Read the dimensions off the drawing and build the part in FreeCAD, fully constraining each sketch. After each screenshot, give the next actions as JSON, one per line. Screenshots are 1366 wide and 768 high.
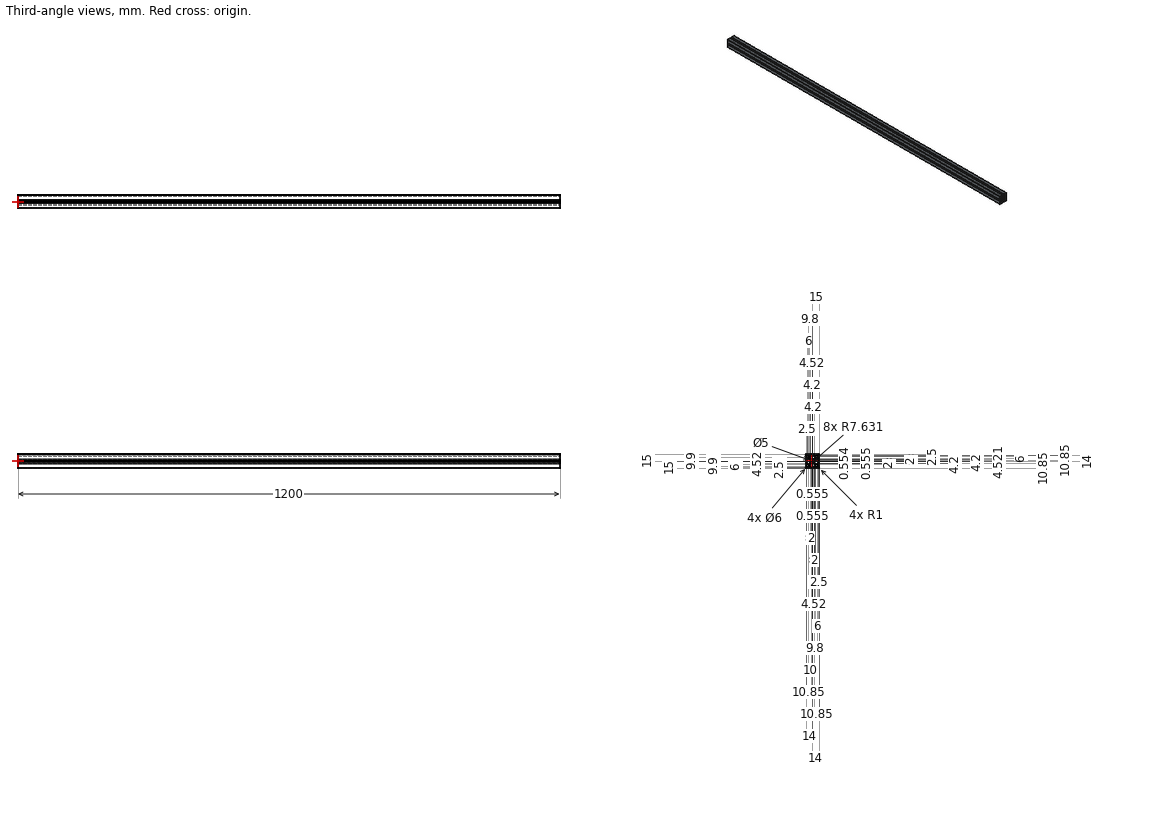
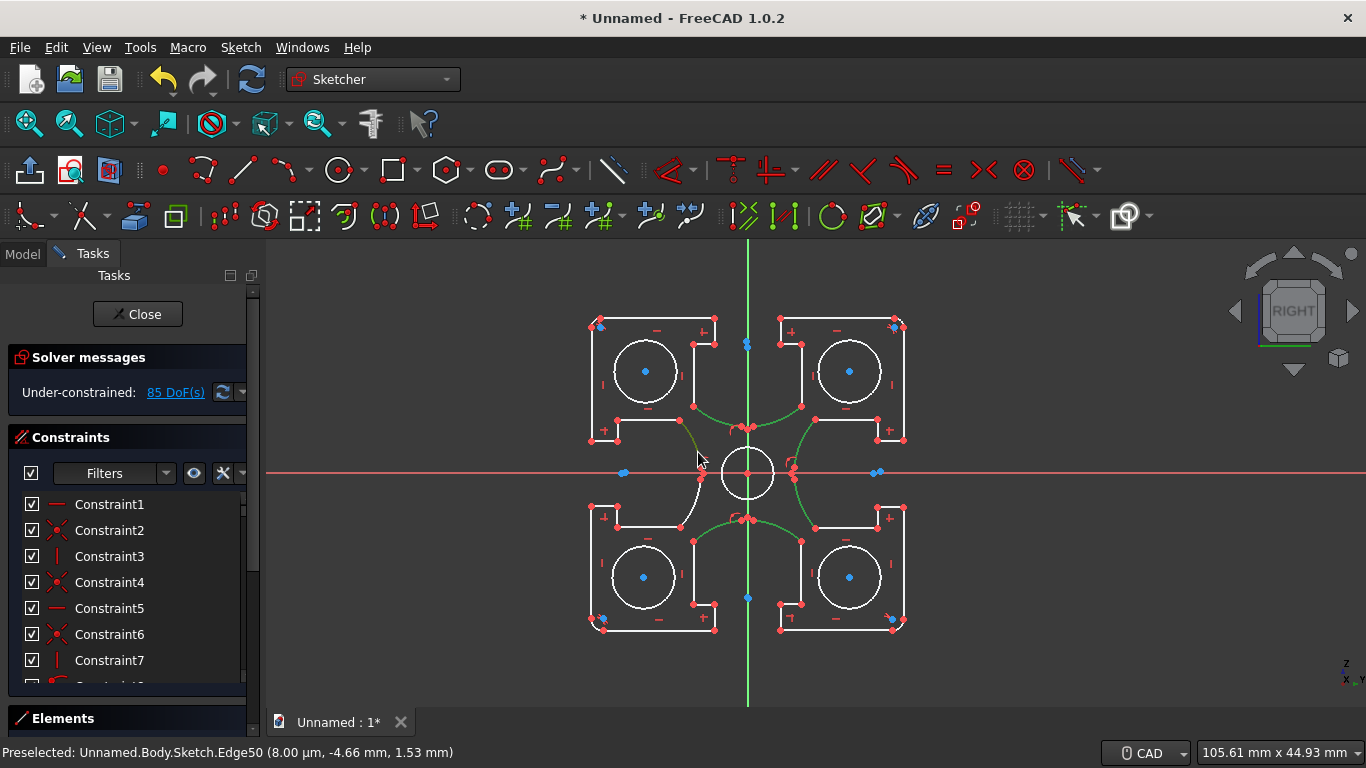
{"action": "left_click", "coordinate": [690, 514]}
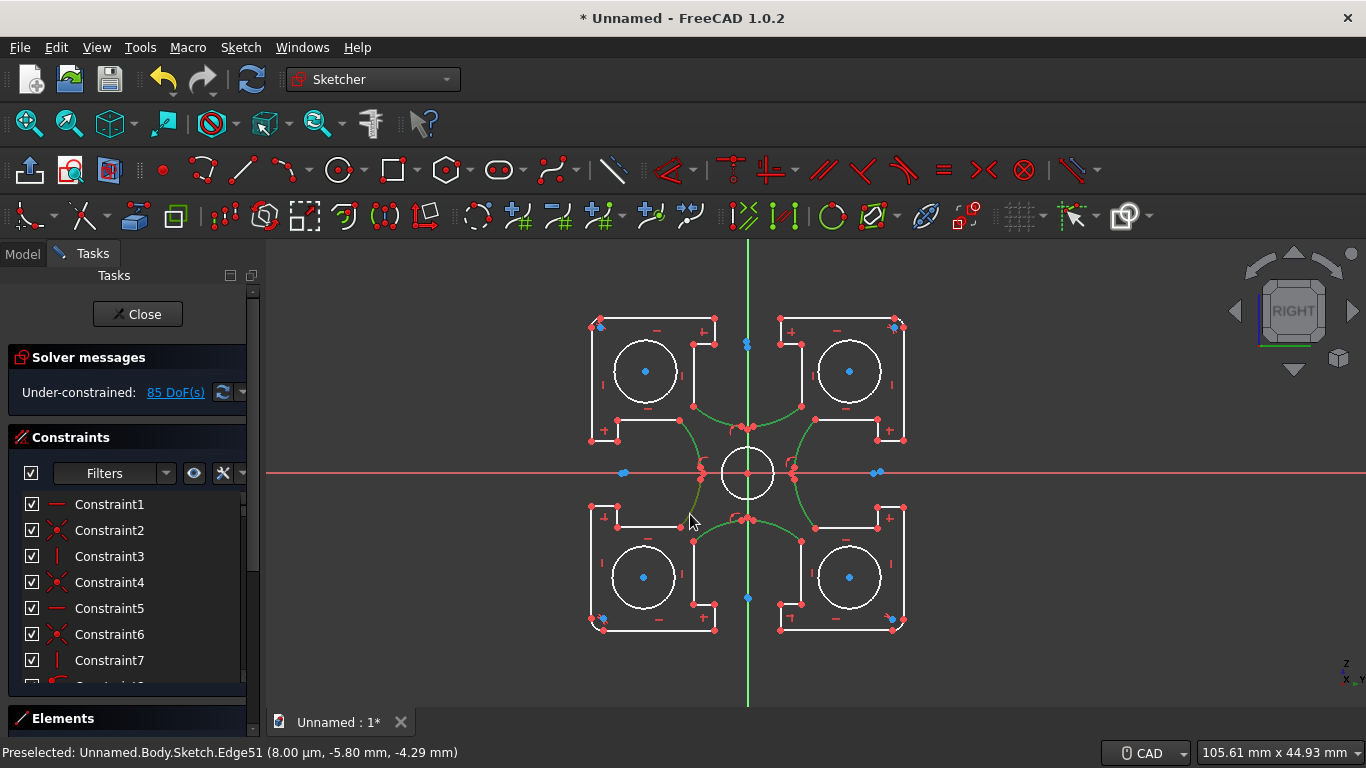
{"action": "left_click", "coordinate": [944, 170]}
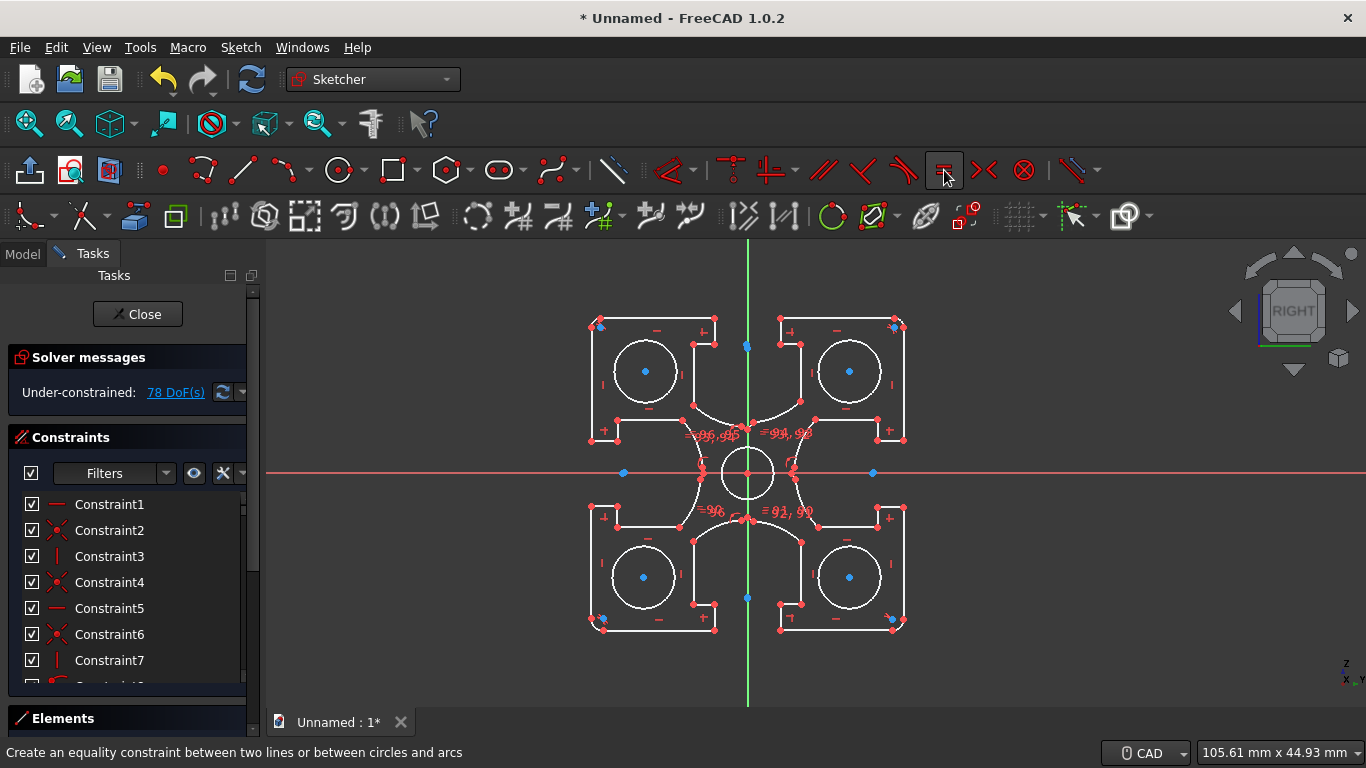
{"action": "scroll", "coordinate": [900, 627], "scroll_direction": "up", "scroll_amount": 3}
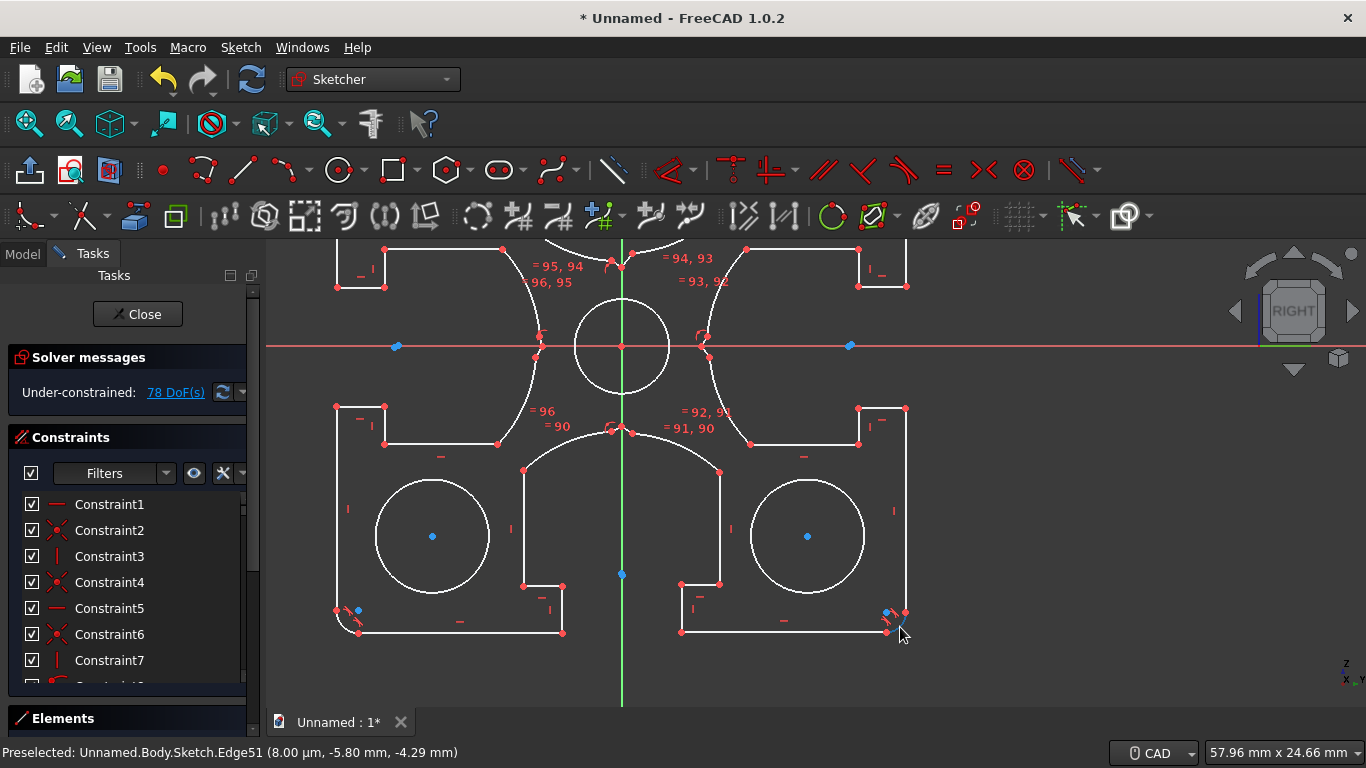
{"action": "left_click", "coordinate": [900, 627]}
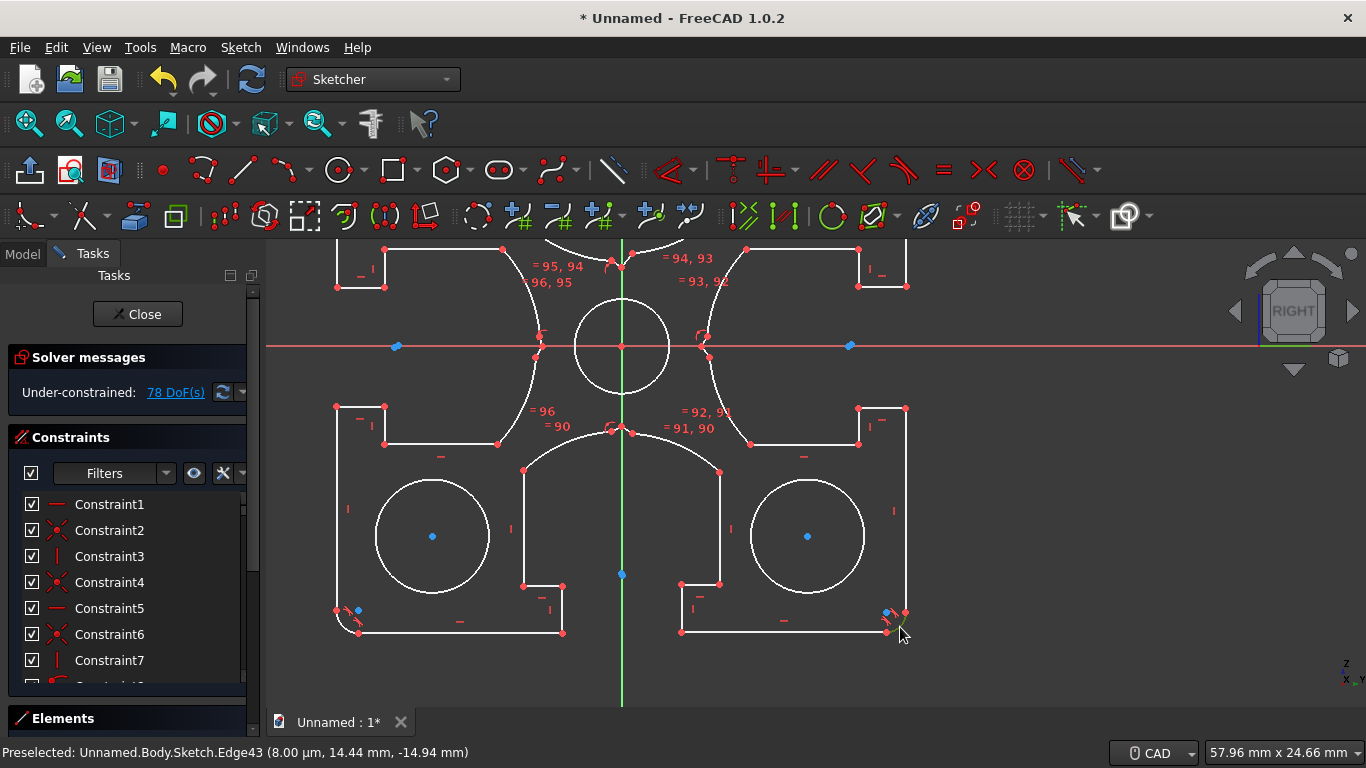
{"action": "scroll", "coordinate": [900, 627], "scroll_direction": "down", "scroll_amount": 3}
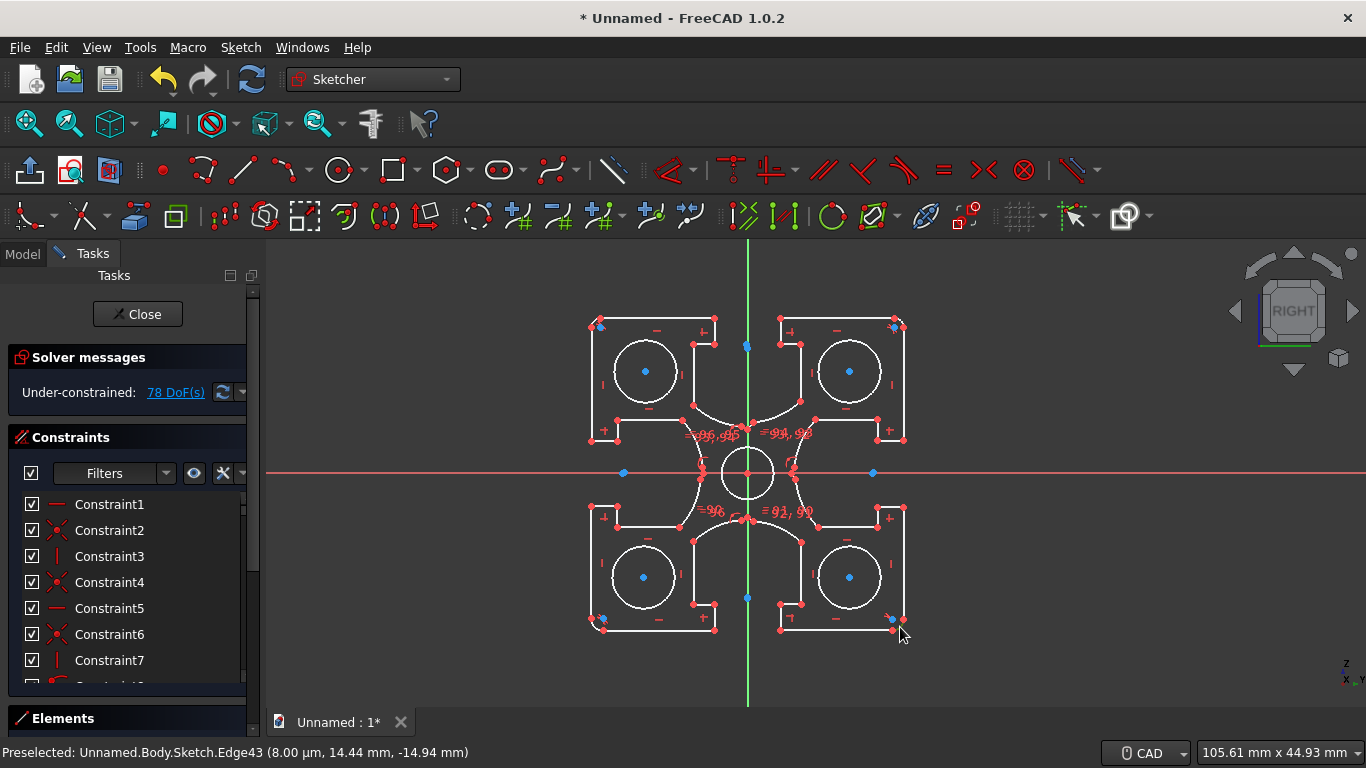
{"action": "scroll", "coordinate": [901, 321], "scroll_direction": "up", "scroll_amount": 4}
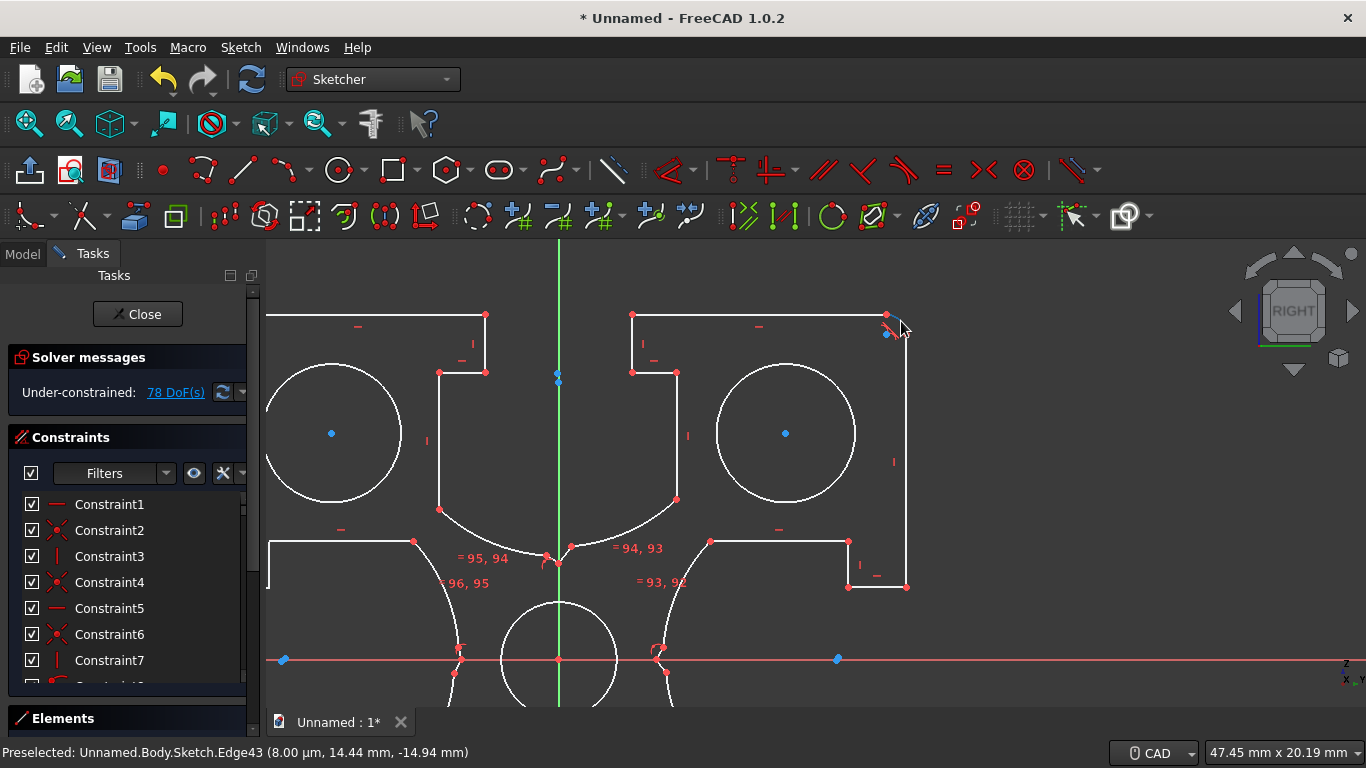
{"action": "left_click", "coordinate": [901, 321]}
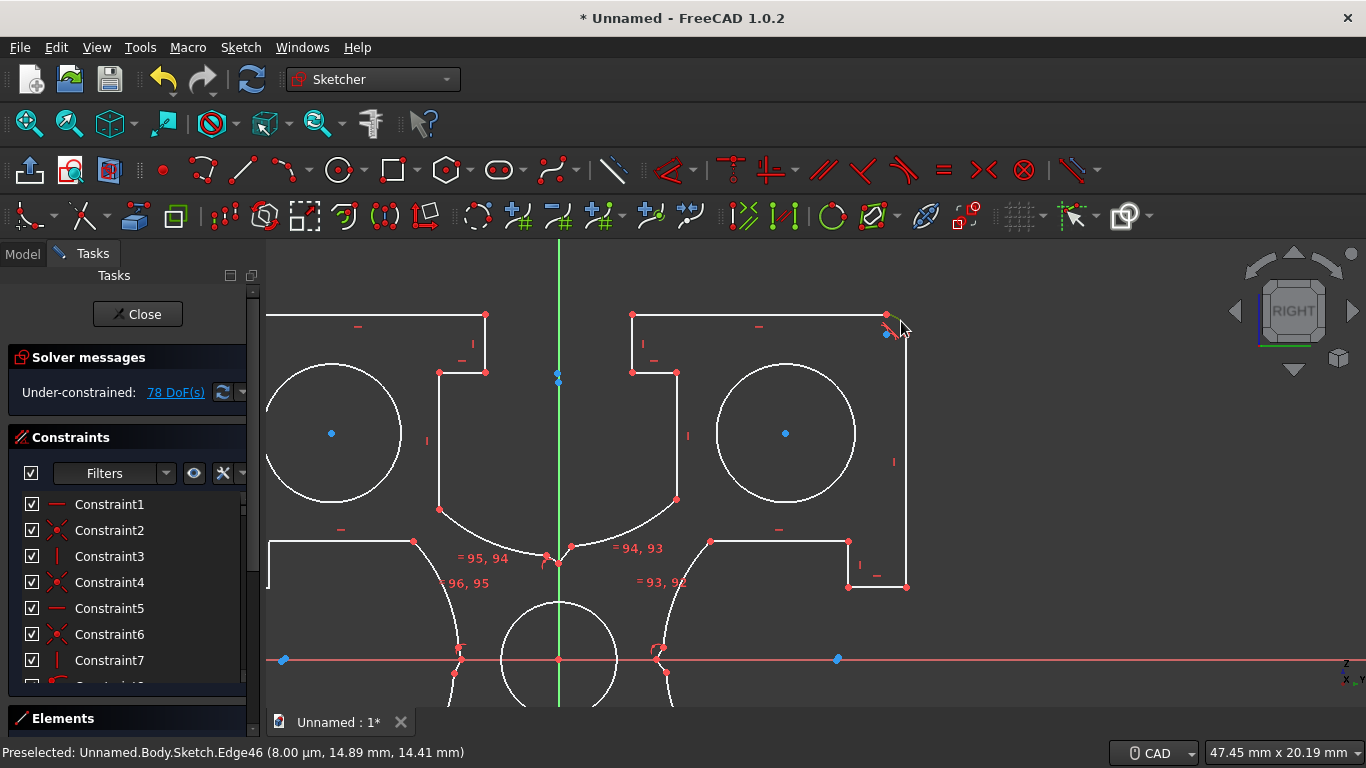
{"action": "scroll", "coordinate": [901, 321], "scroll_direction": "down", "scroll_amount": 4}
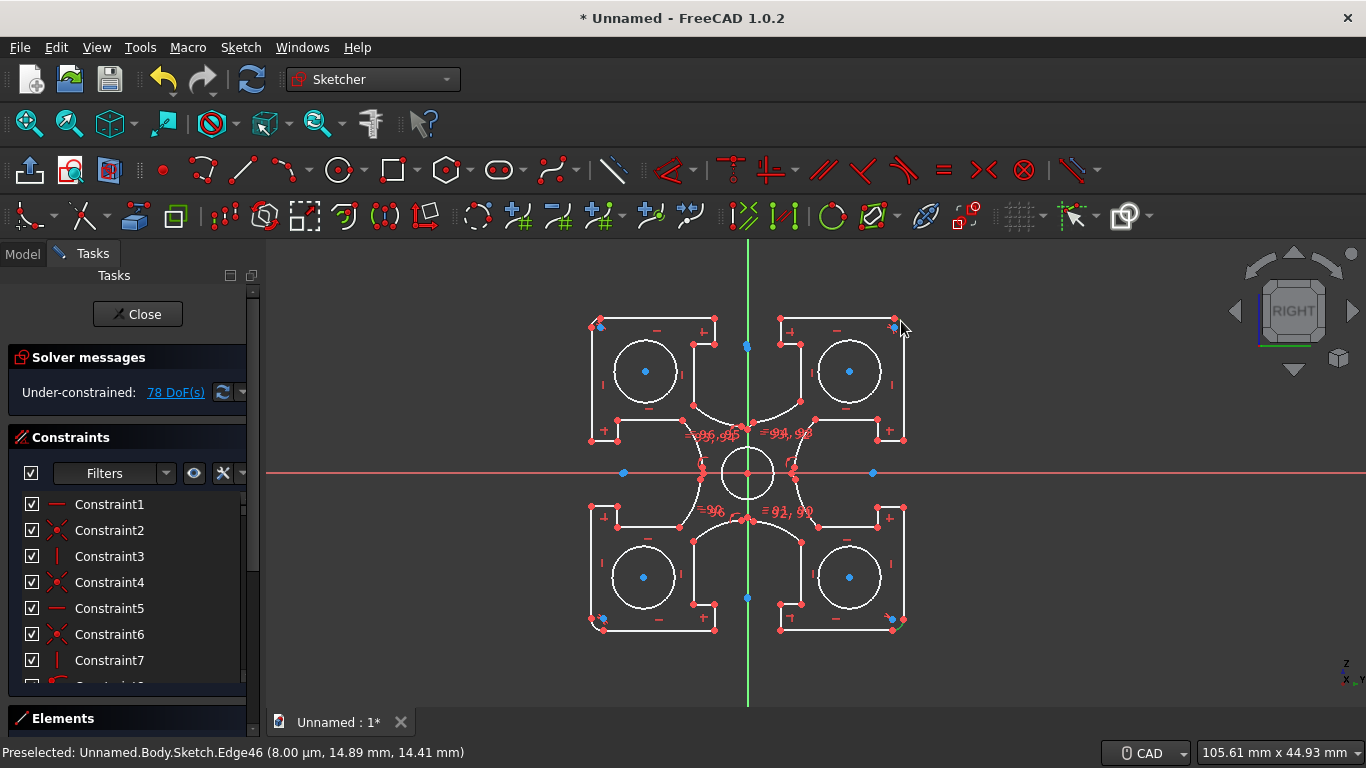
{"action": "scroll", "coordinate": [596, 319], "scroll_direction": "up", "scroll_amount": 7}